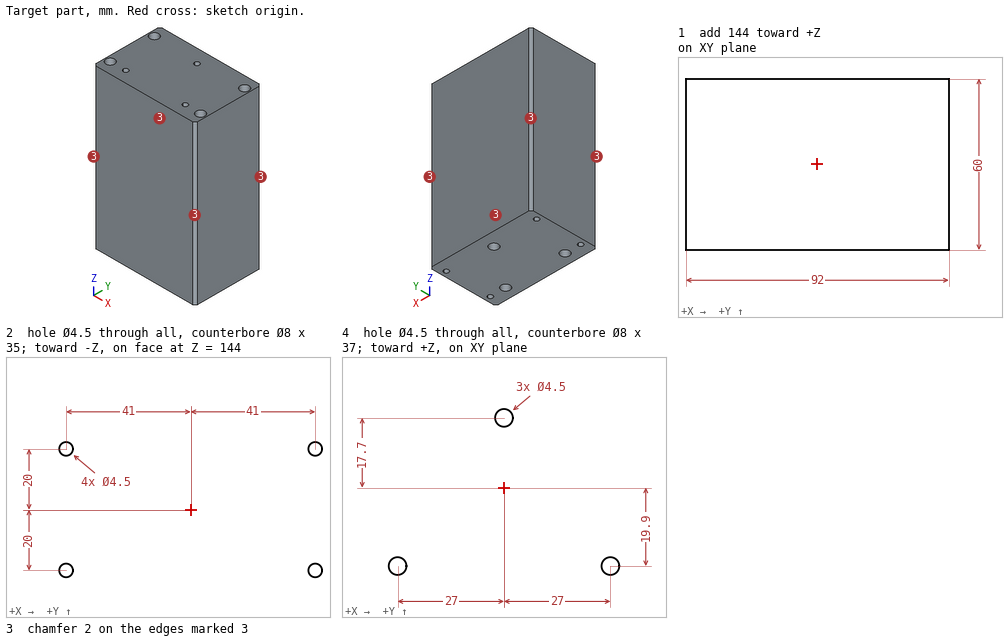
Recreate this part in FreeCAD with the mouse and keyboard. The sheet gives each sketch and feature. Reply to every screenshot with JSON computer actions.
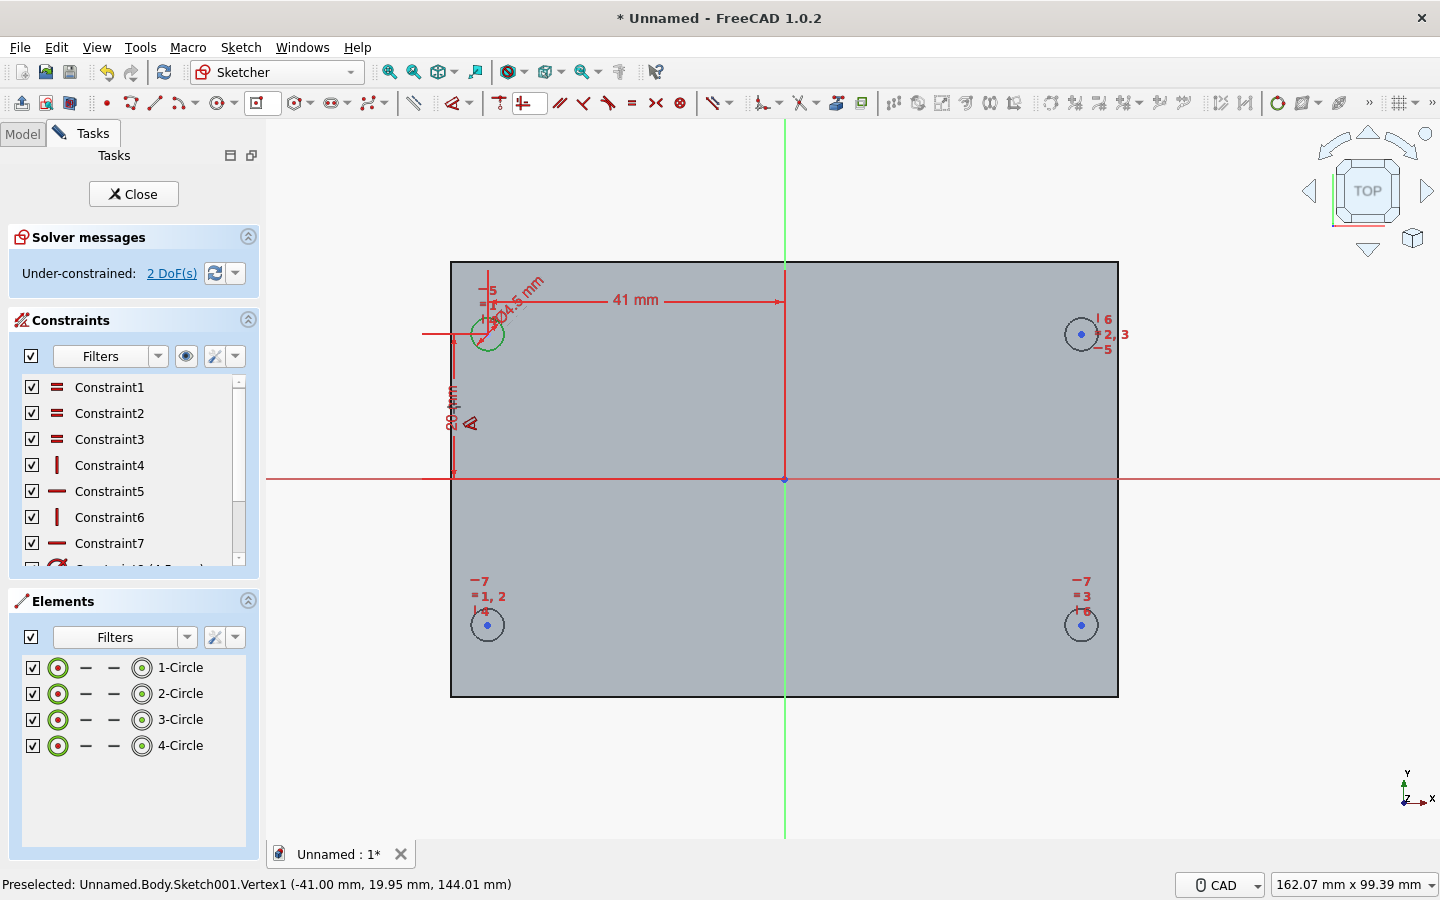
{"action": "left_click", "coordinate": [488, 625]}
{"action": "left_click", "coordinate": [454, 552]}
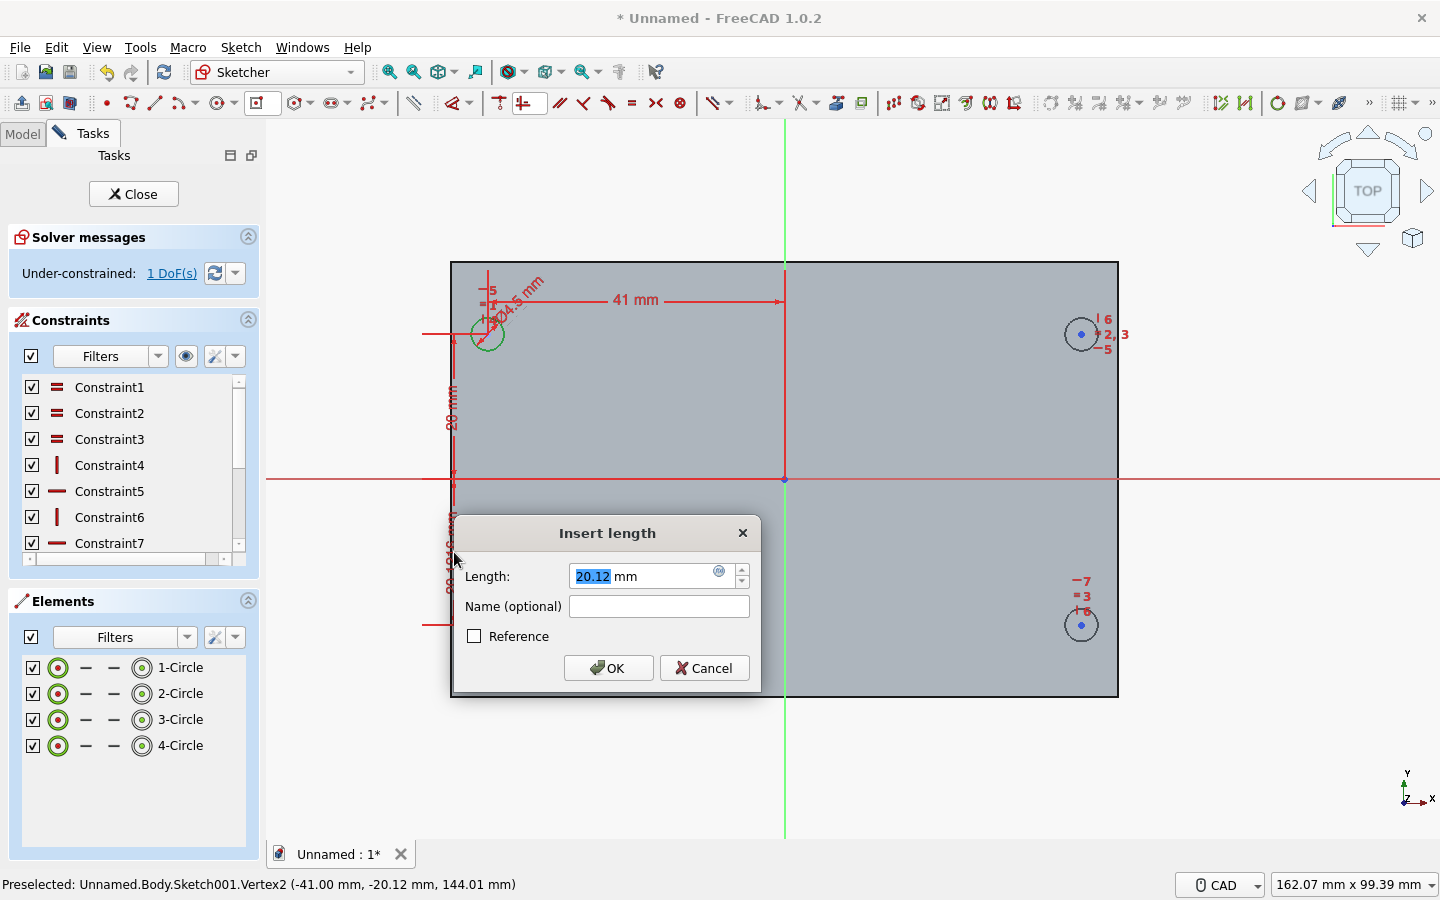
{"action": "type", "text": "20"}
{"action": "key", "text": "Return"}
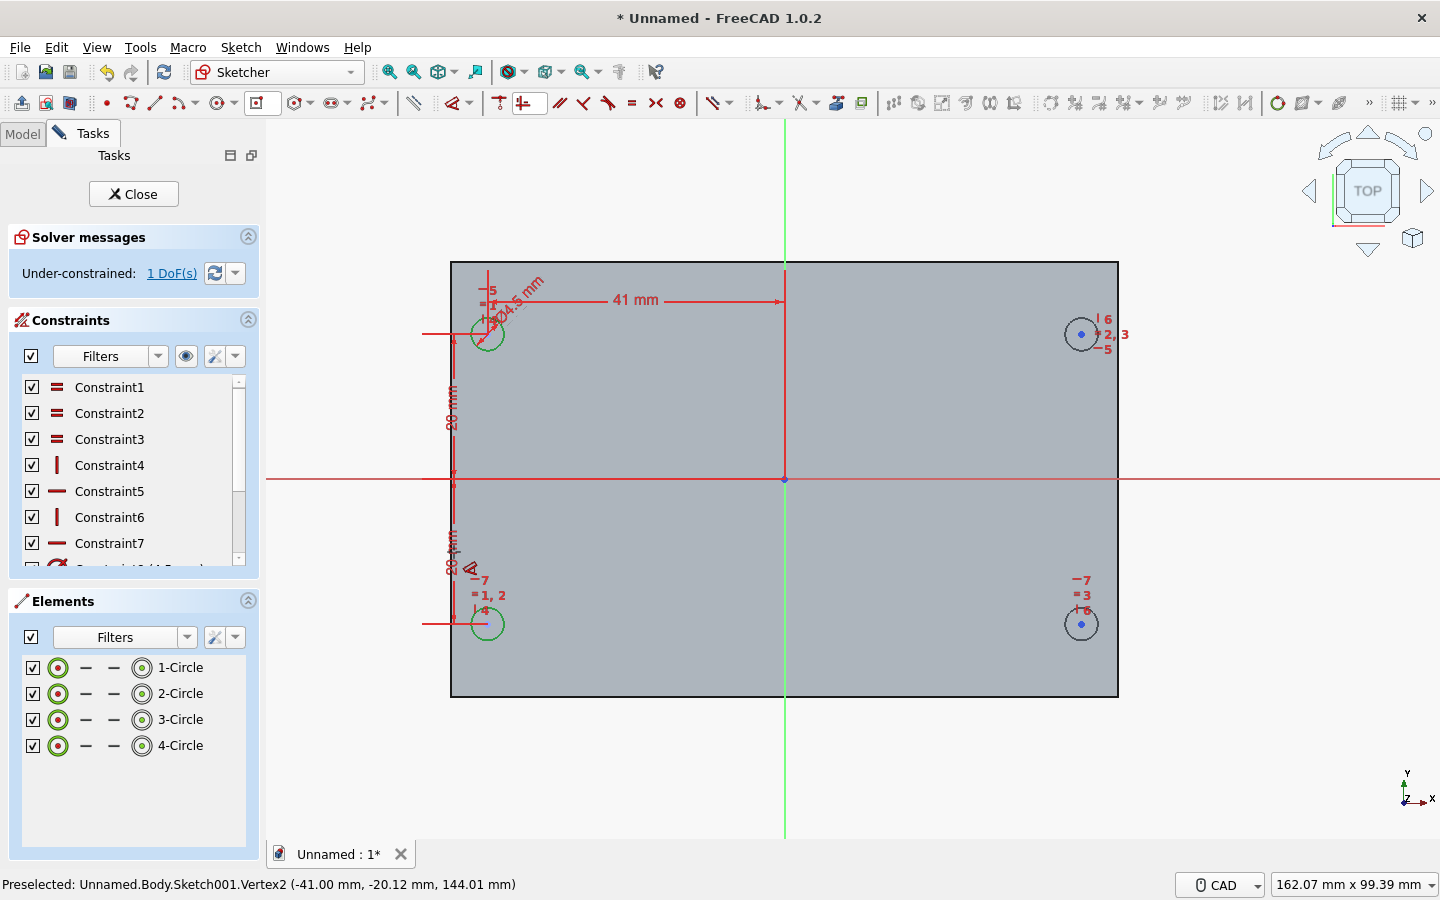
{"action": "left_click", "coordinate": [1082, 334]}
{"action": "left_click", "coordinate": [933, 300]}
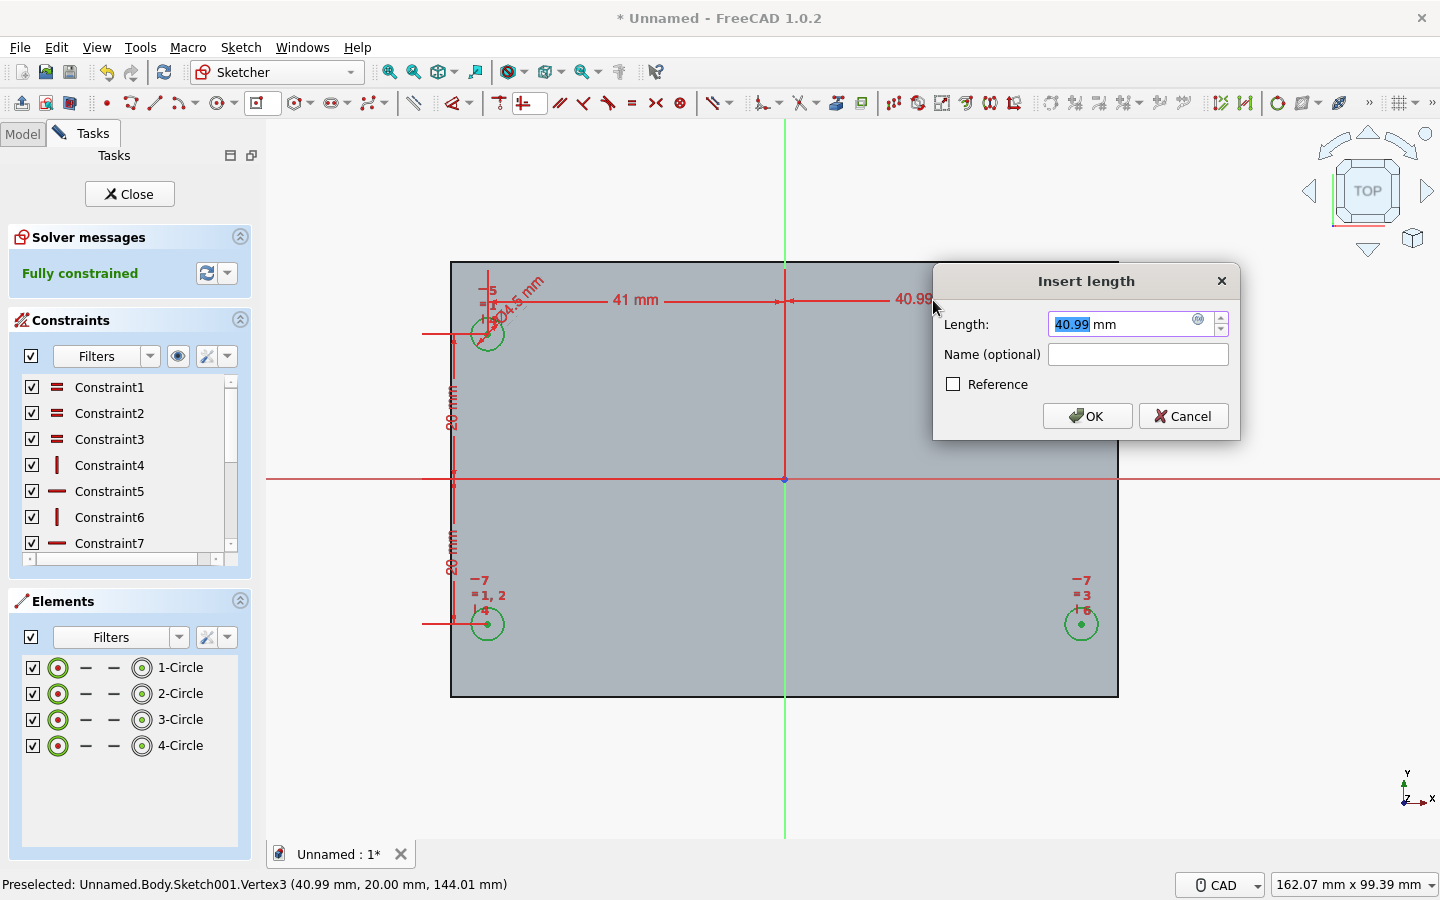
{"action": "type", "text": "41"}
{"action": "key", "text": "Return"}
{"action": "key", "text": "Escape"}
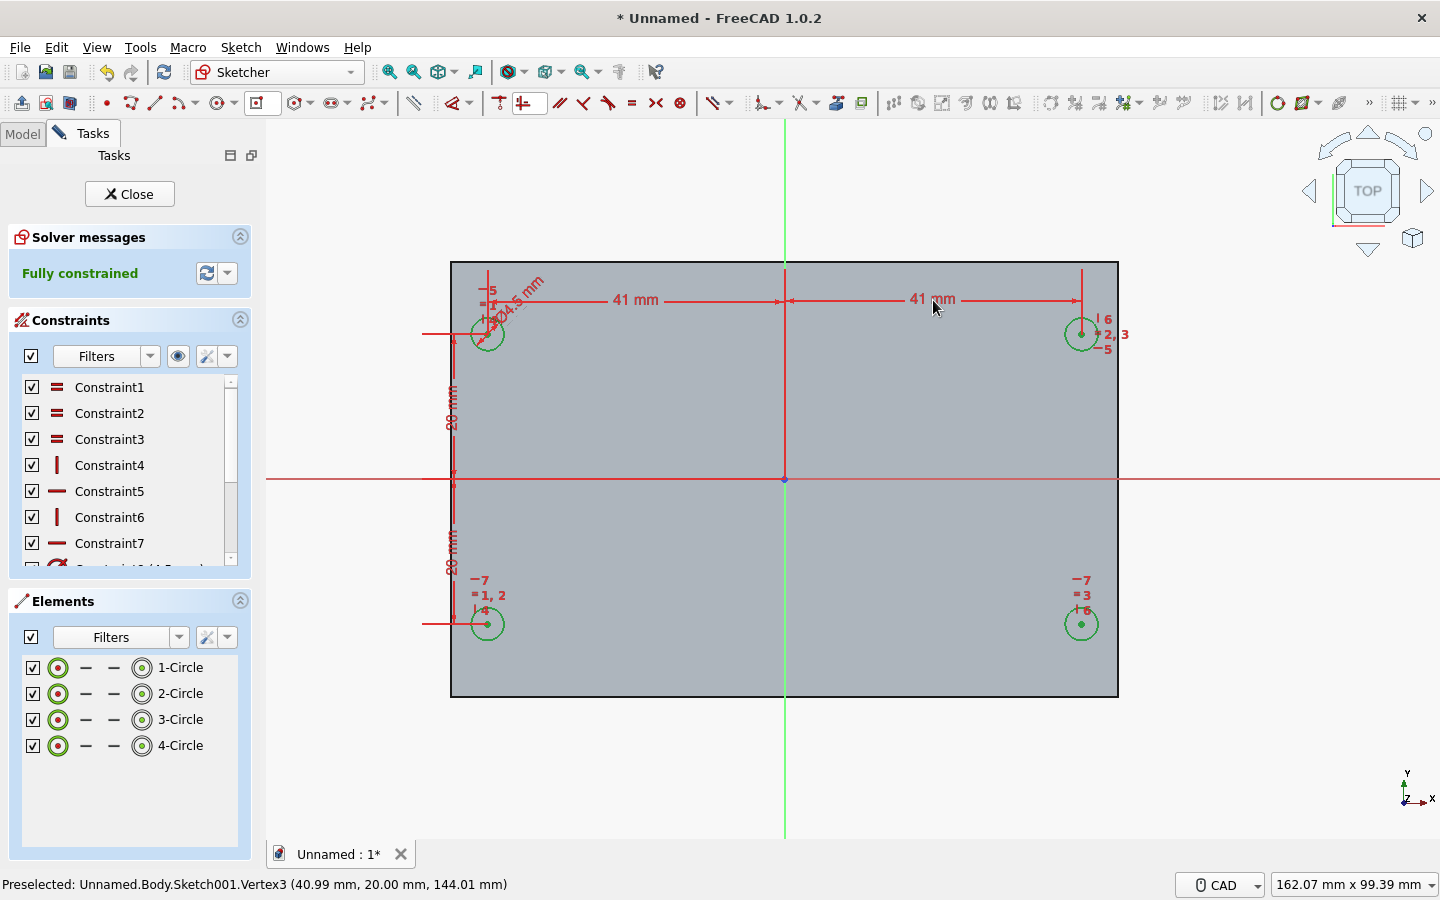
{"action": "left_click", "coordinate": [130, 194]}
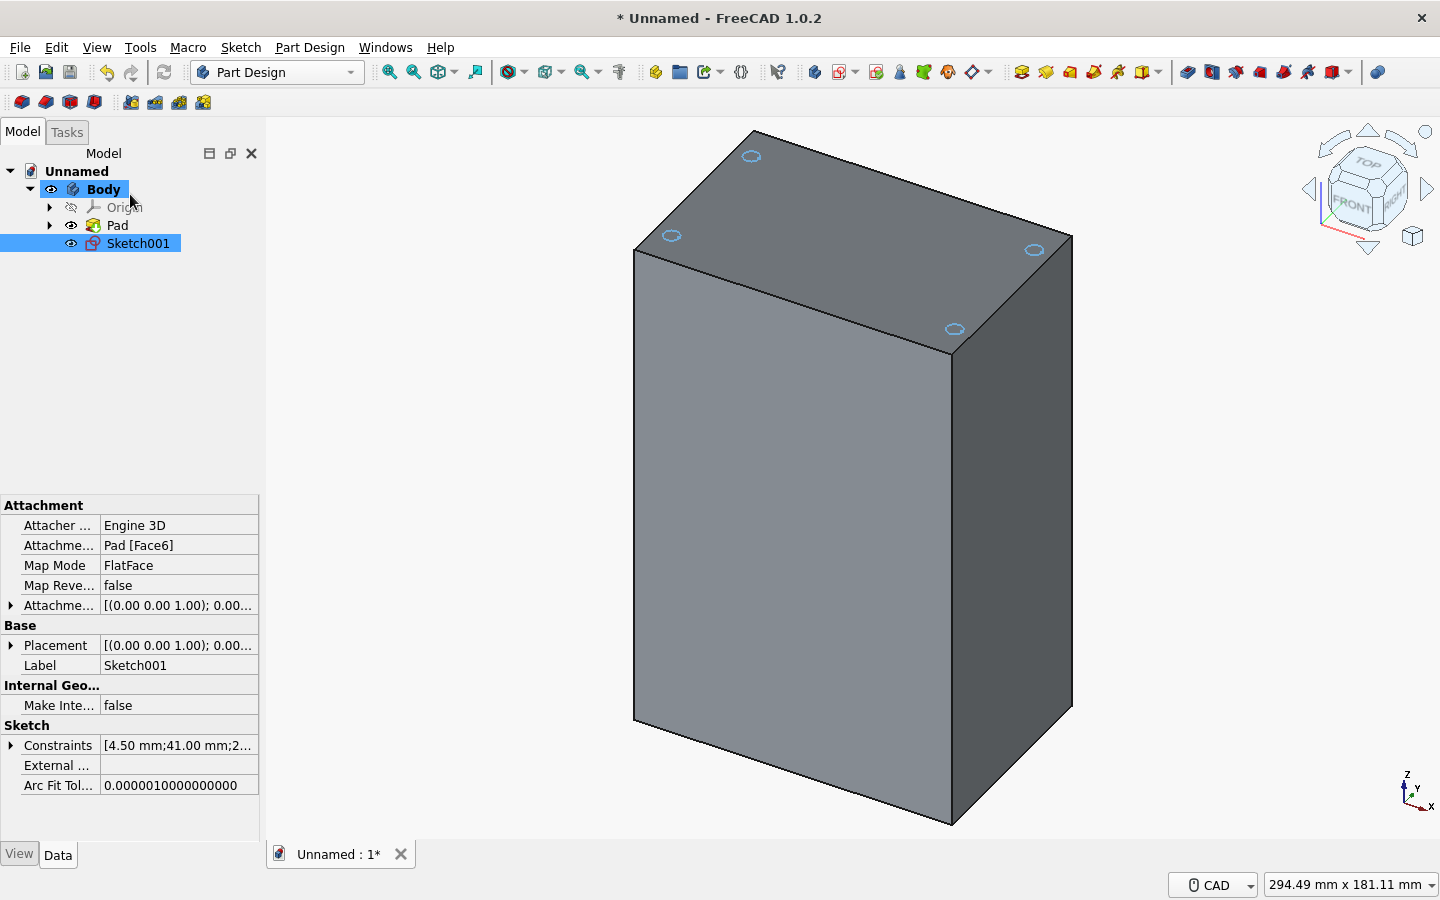
{"action": "left_click", "coordinate": [1212, 72]}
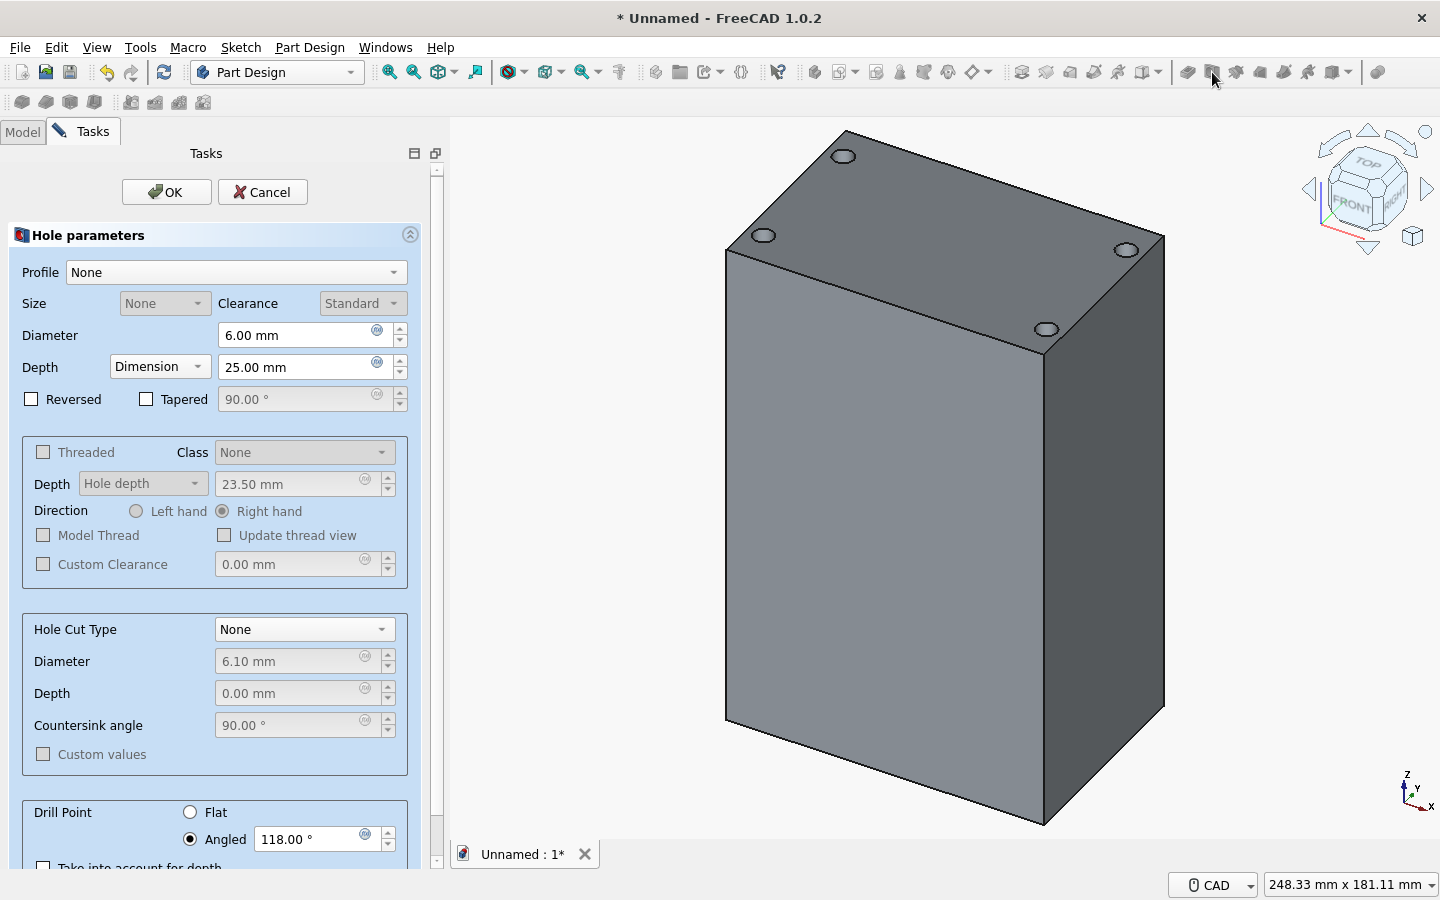
{"action": "triple_click", "coordinate": [305, 335]}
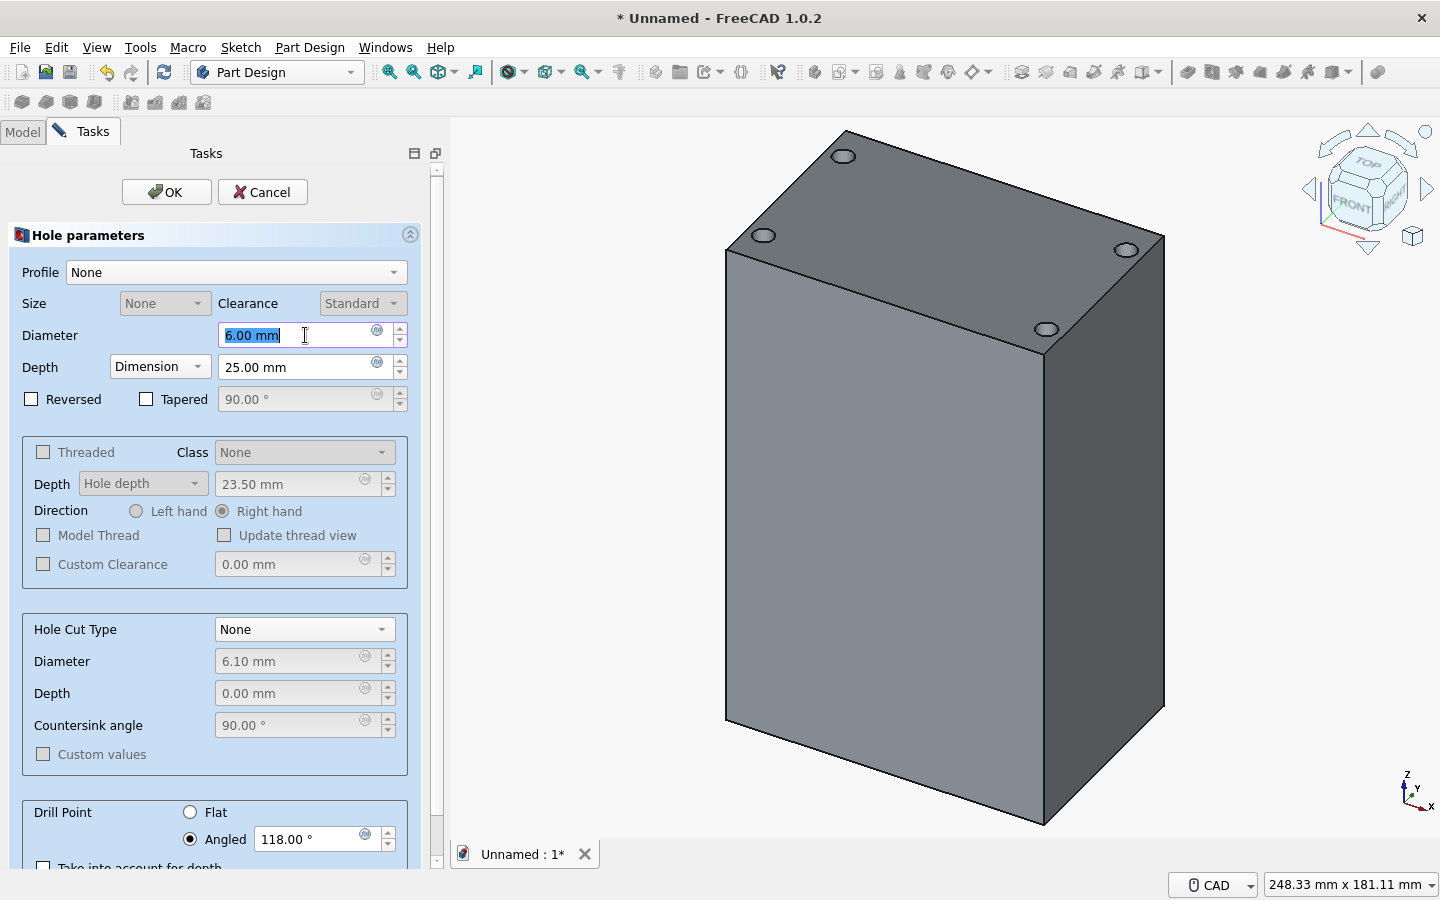
{"action": "type", "text": "4.5"}
{"action": "key", "text": "Tab"}